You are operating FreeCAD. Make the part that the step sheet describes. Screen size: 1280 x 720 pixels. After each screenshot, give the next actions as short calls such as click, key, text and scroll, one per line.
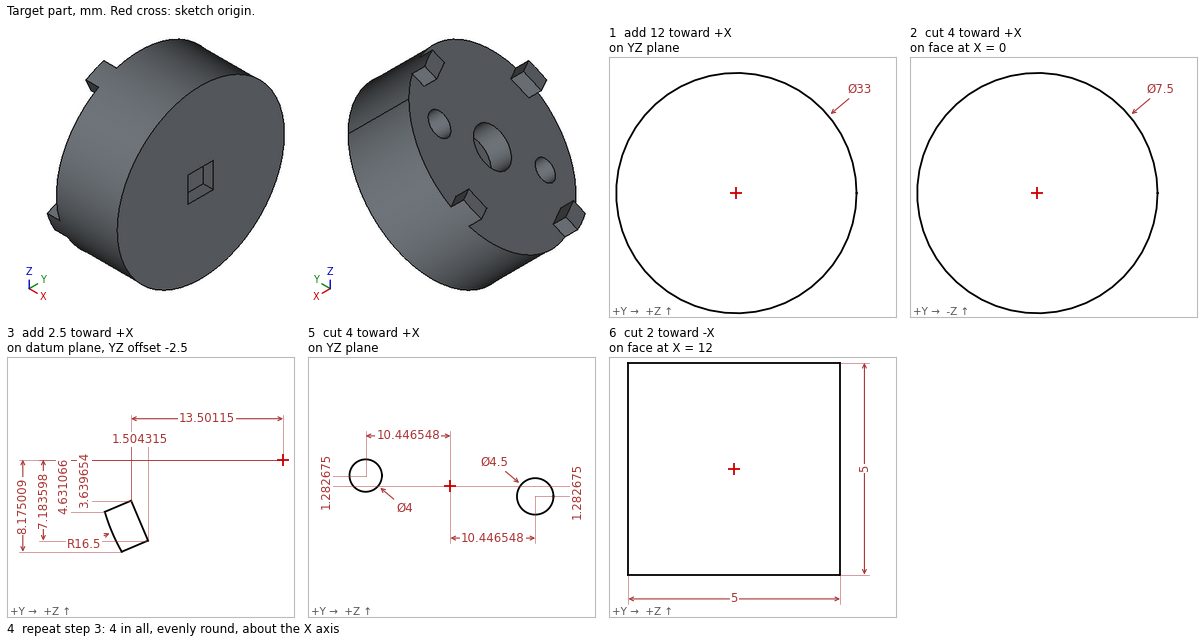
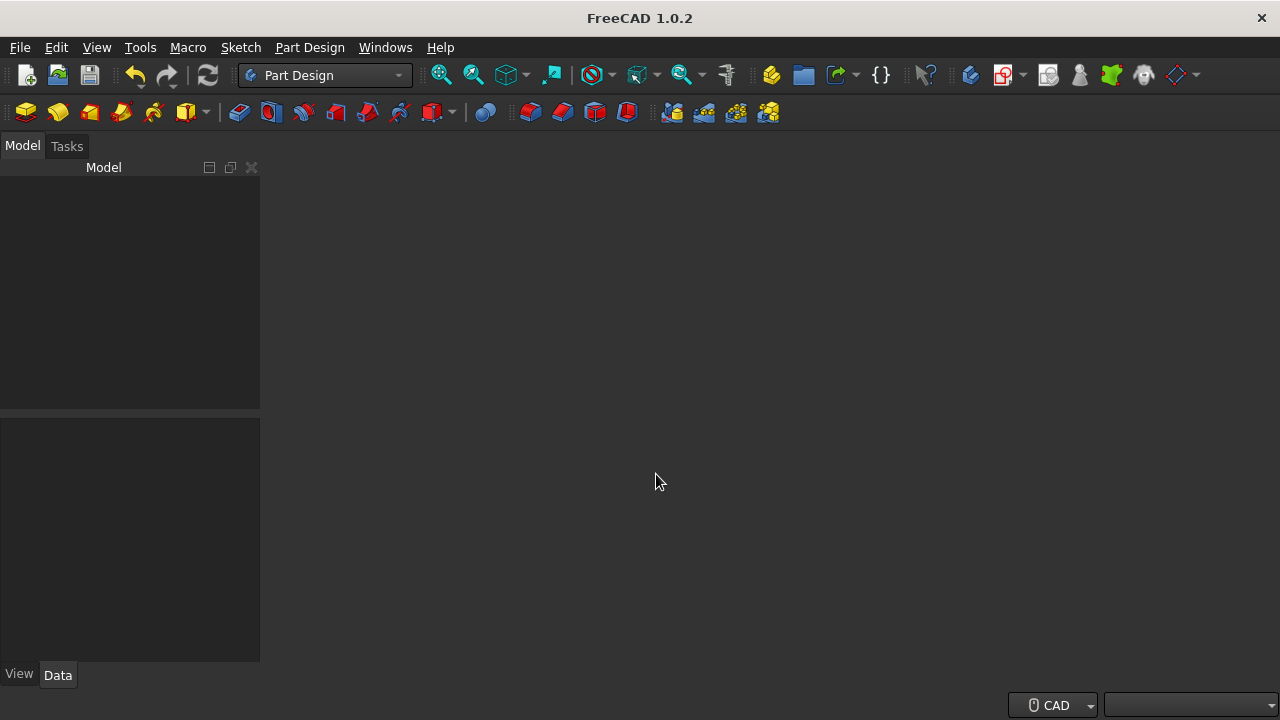
key(ctrl+n)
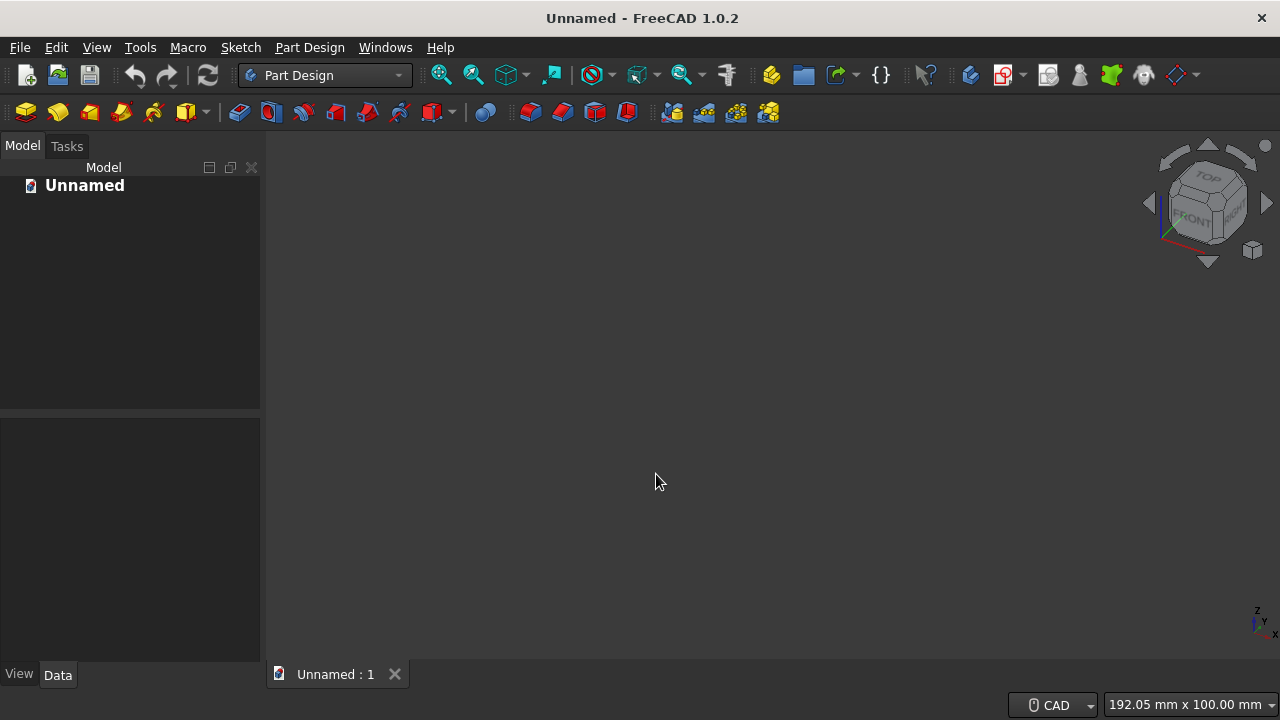
click(1004, 76)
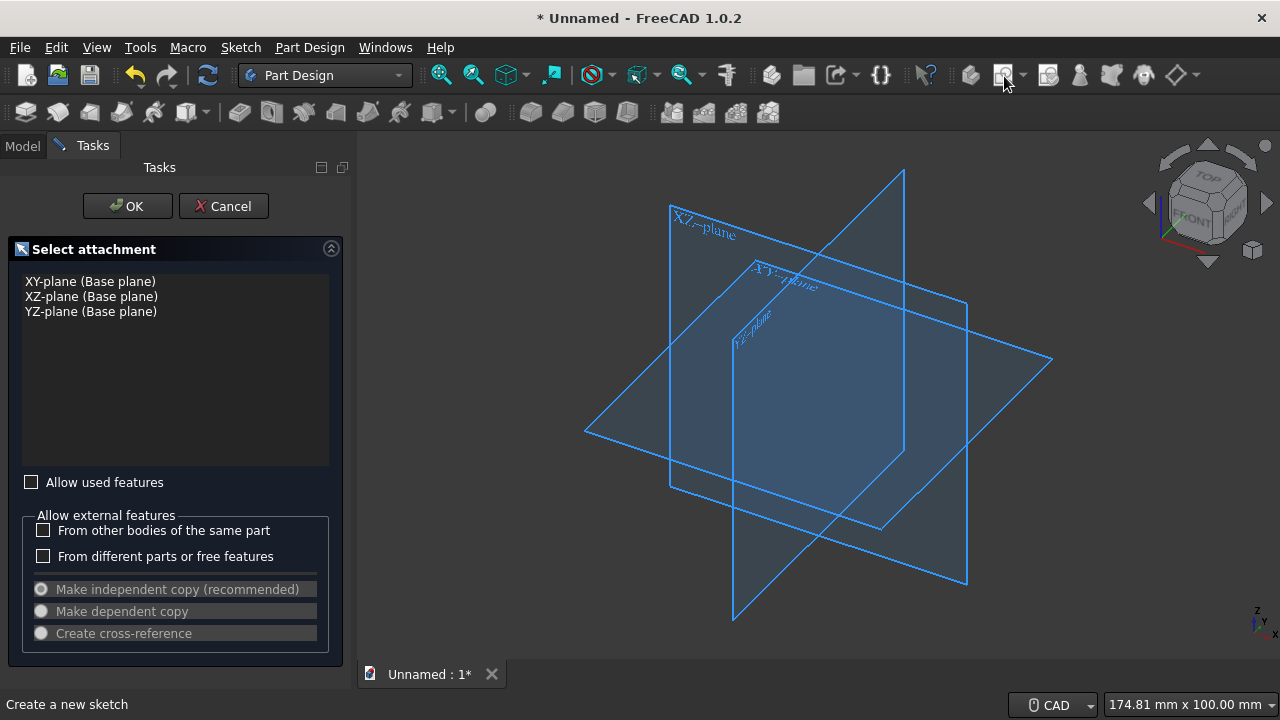
click(82, 312)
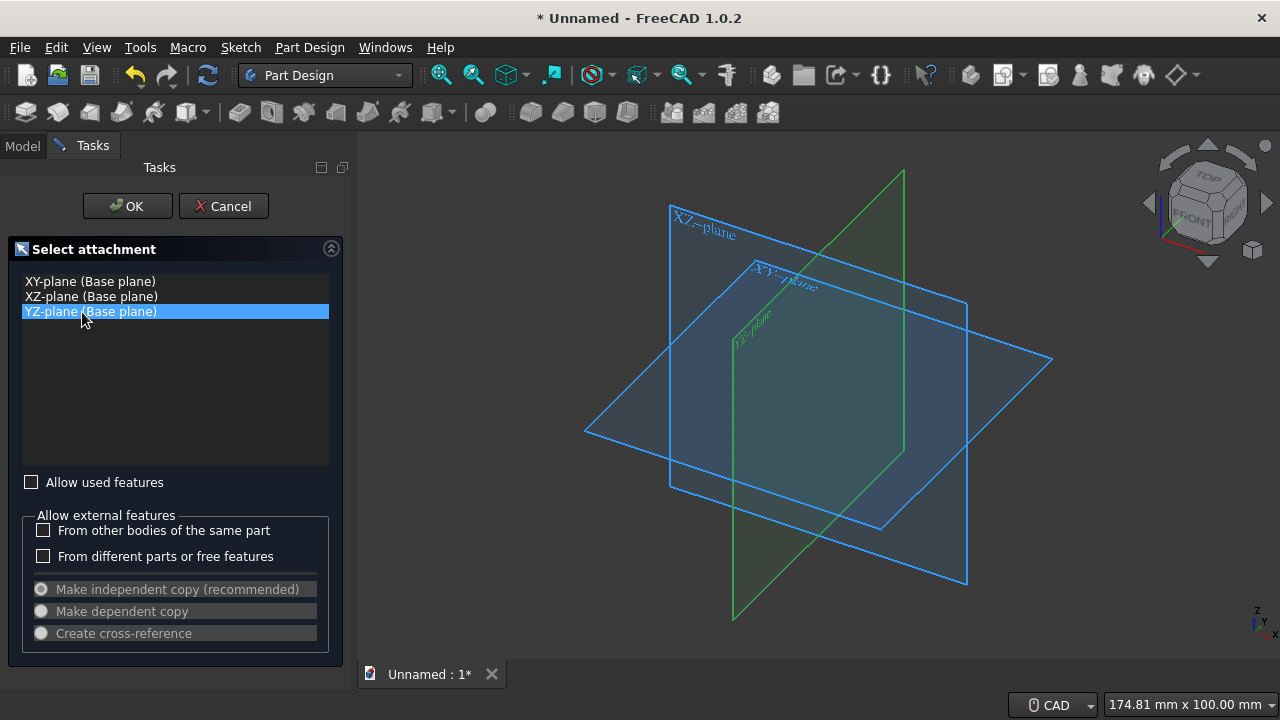
click(128, 206)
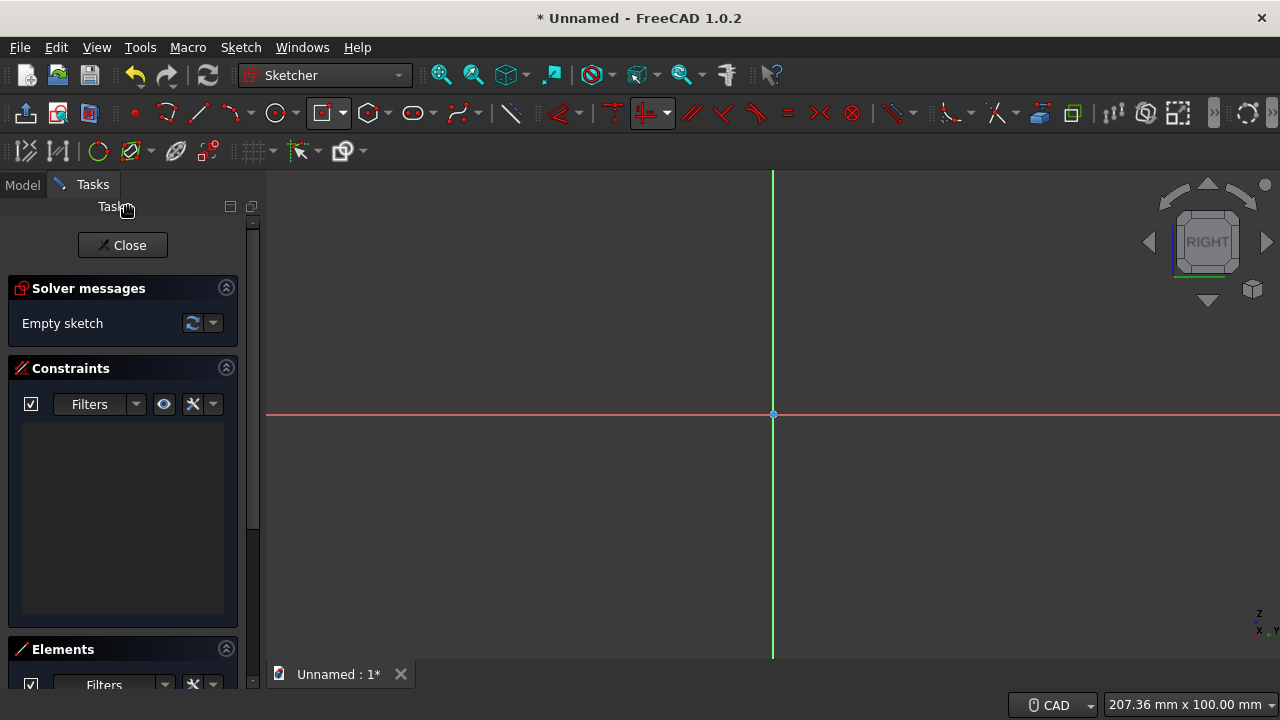
scroll(856, 415, up, 3)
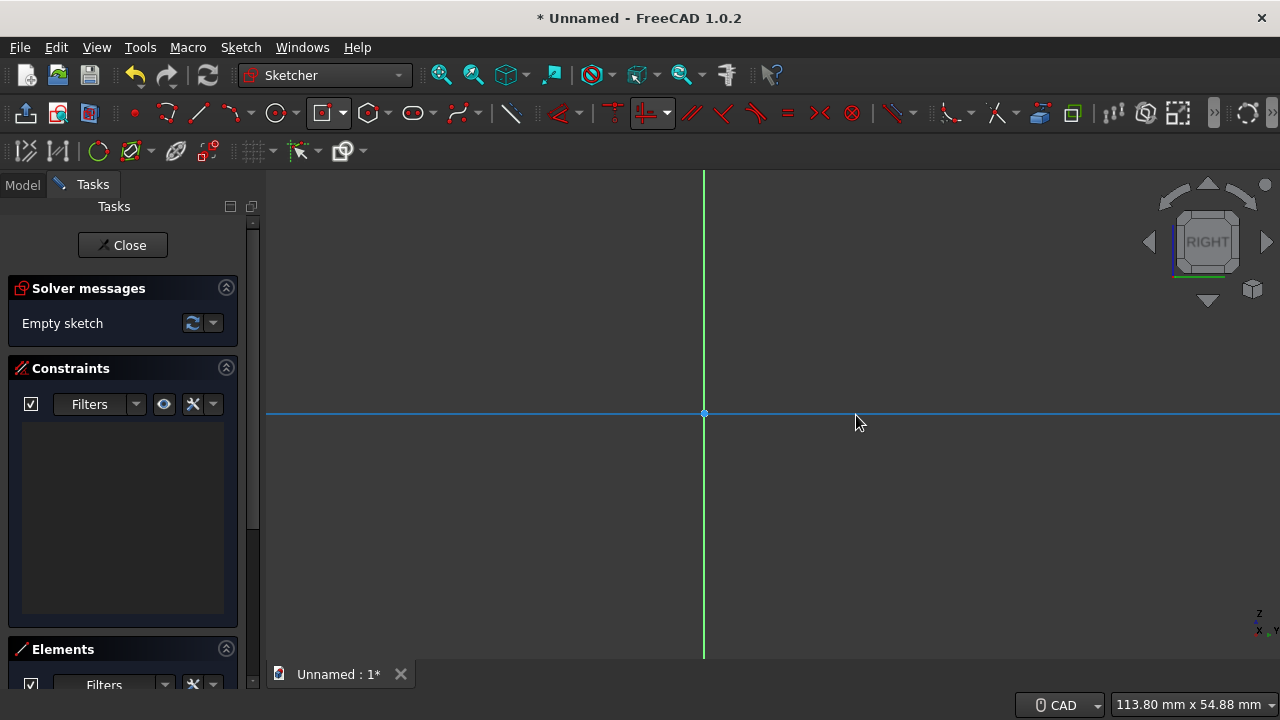
click(276, 114)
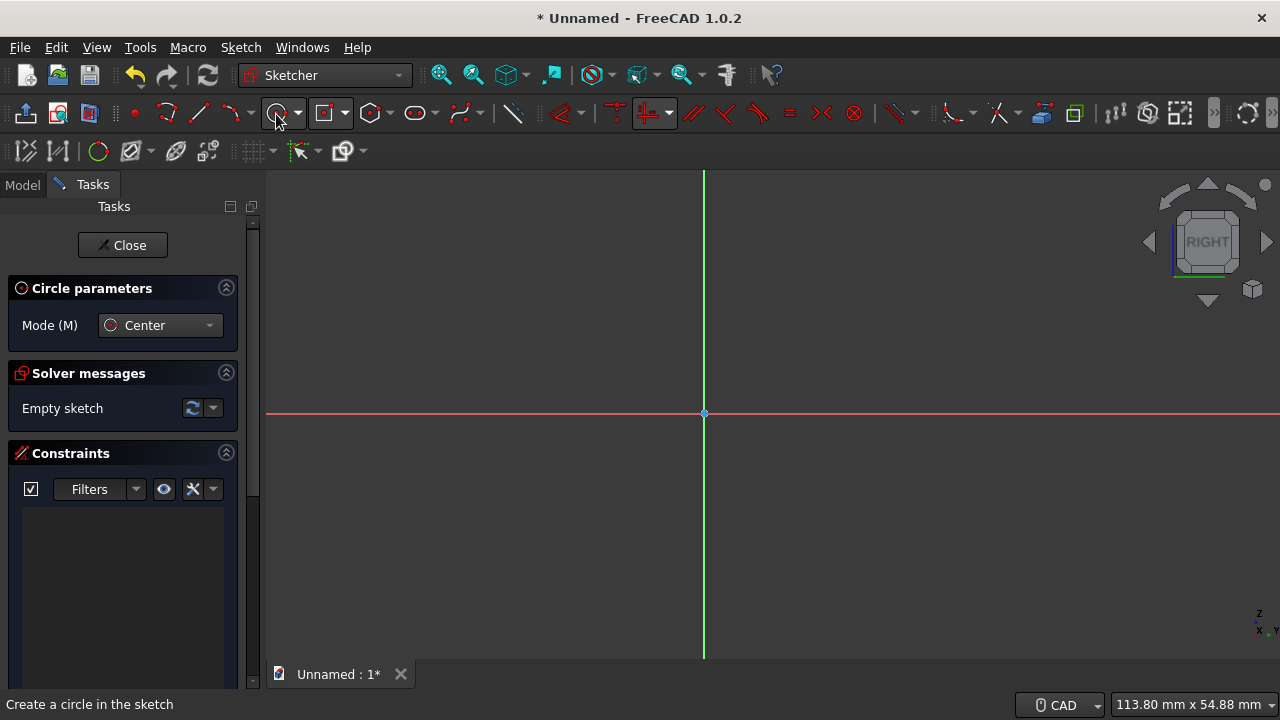
click(704, 414)
click(808, 310)
key(Escape)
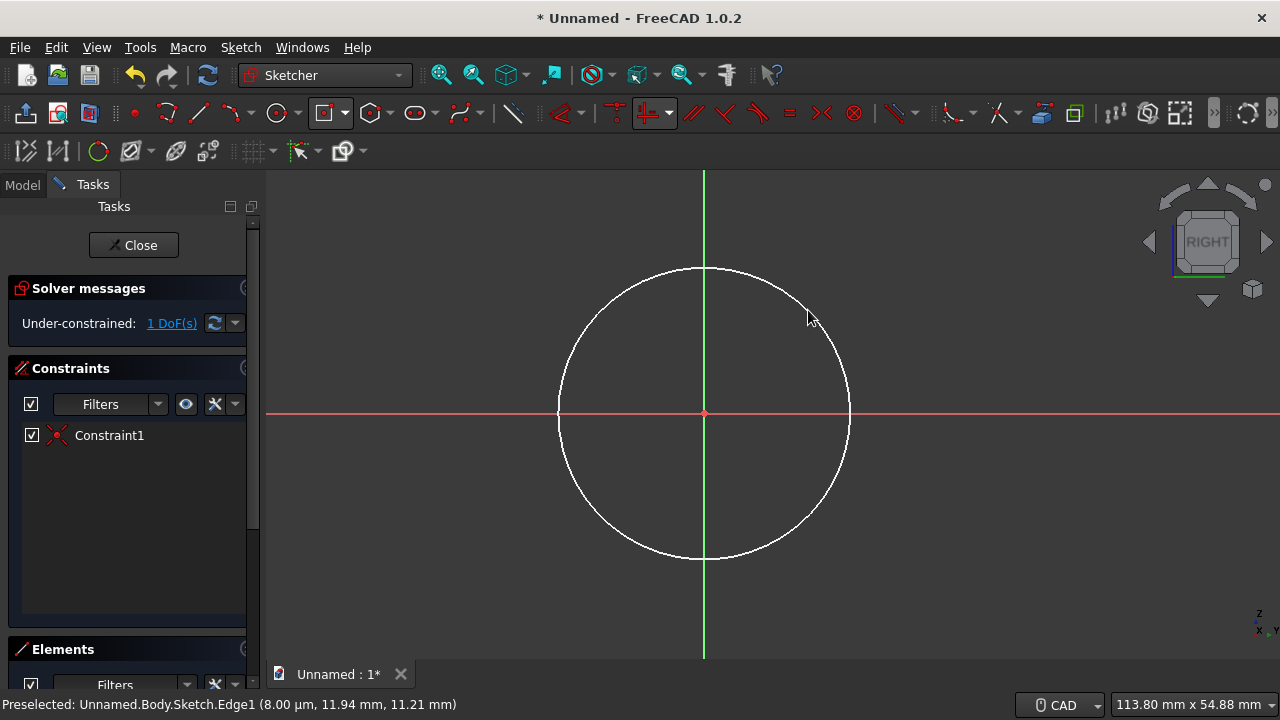
key(d)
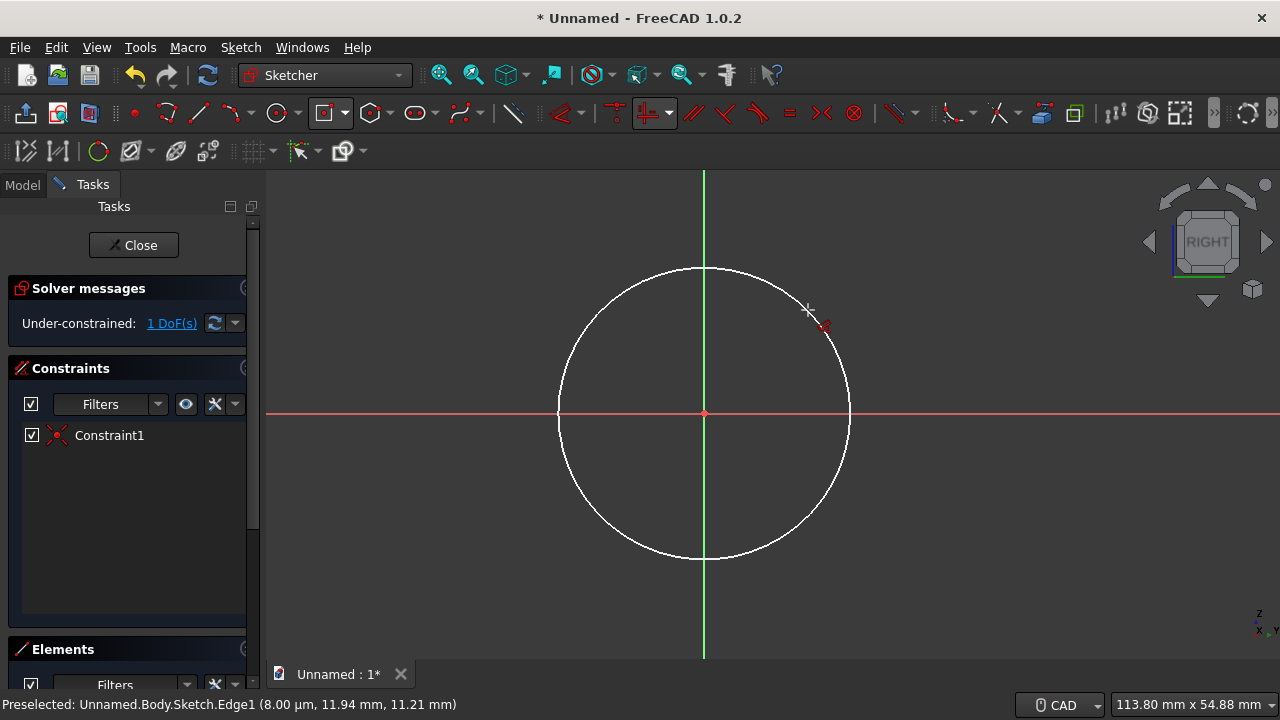
click(807, 310)
click(830, 287)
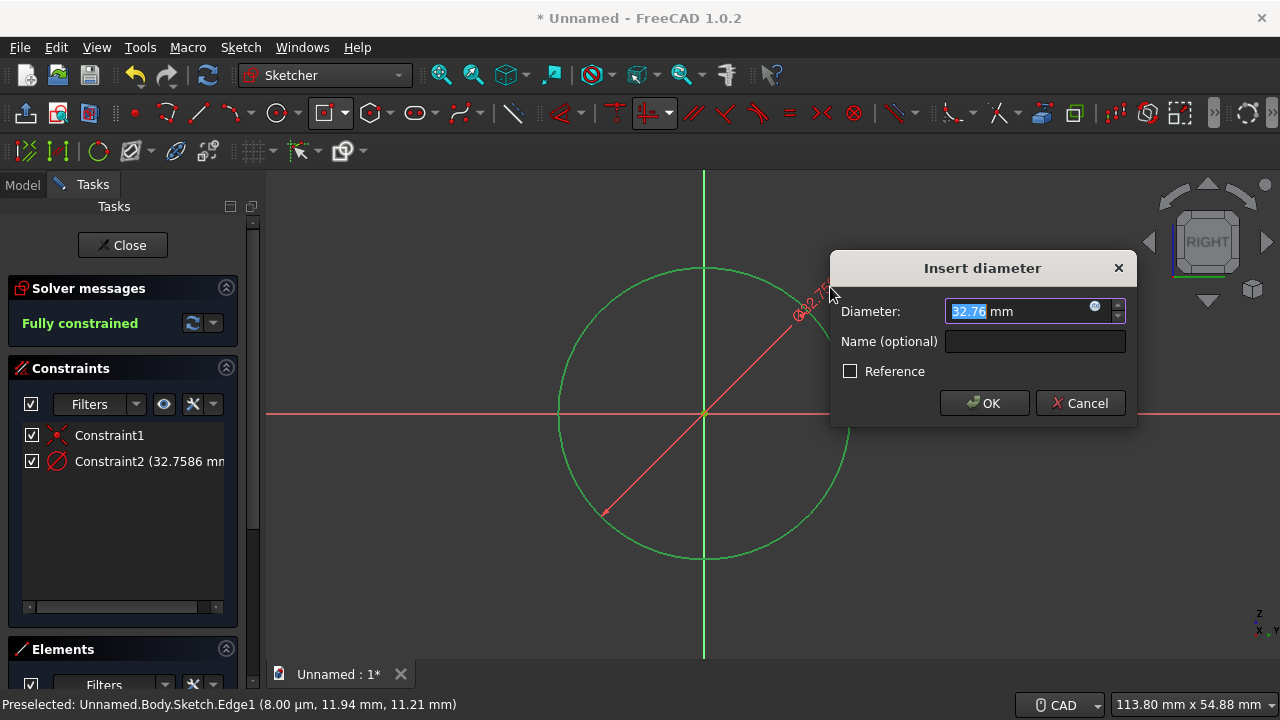
text(33)
key(Return)
key(Escape)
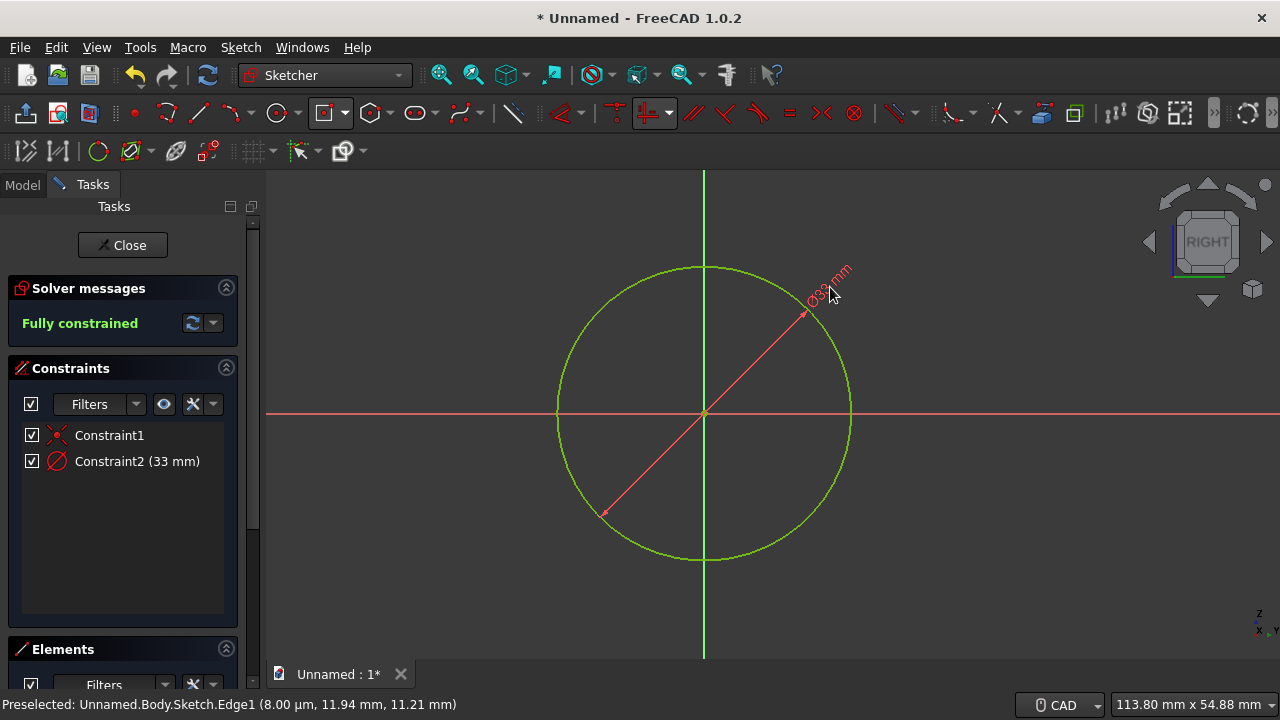
click(123, 245)